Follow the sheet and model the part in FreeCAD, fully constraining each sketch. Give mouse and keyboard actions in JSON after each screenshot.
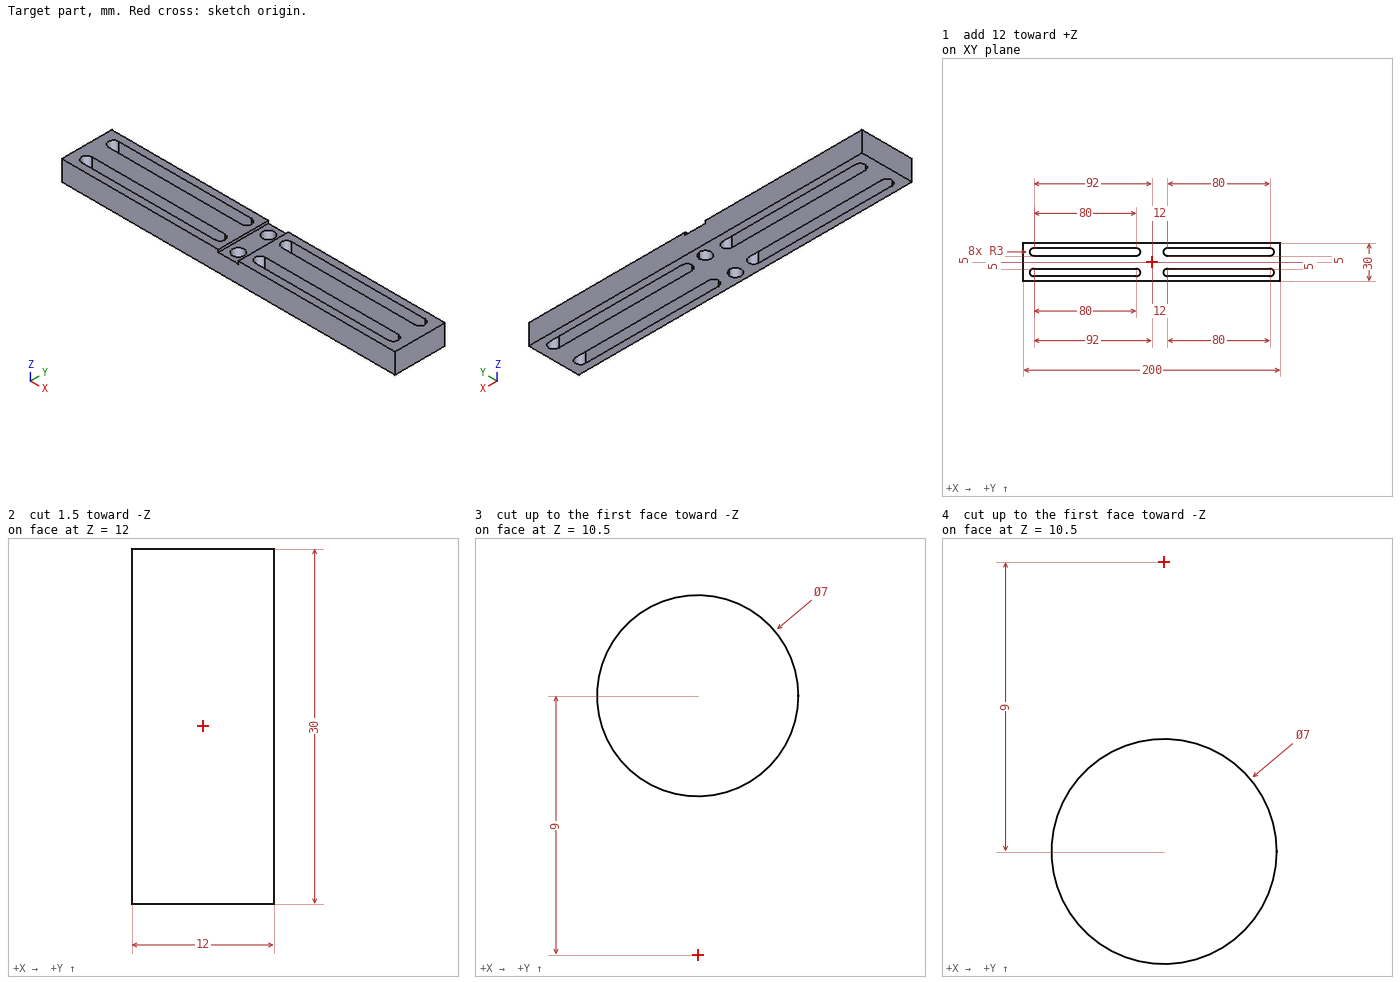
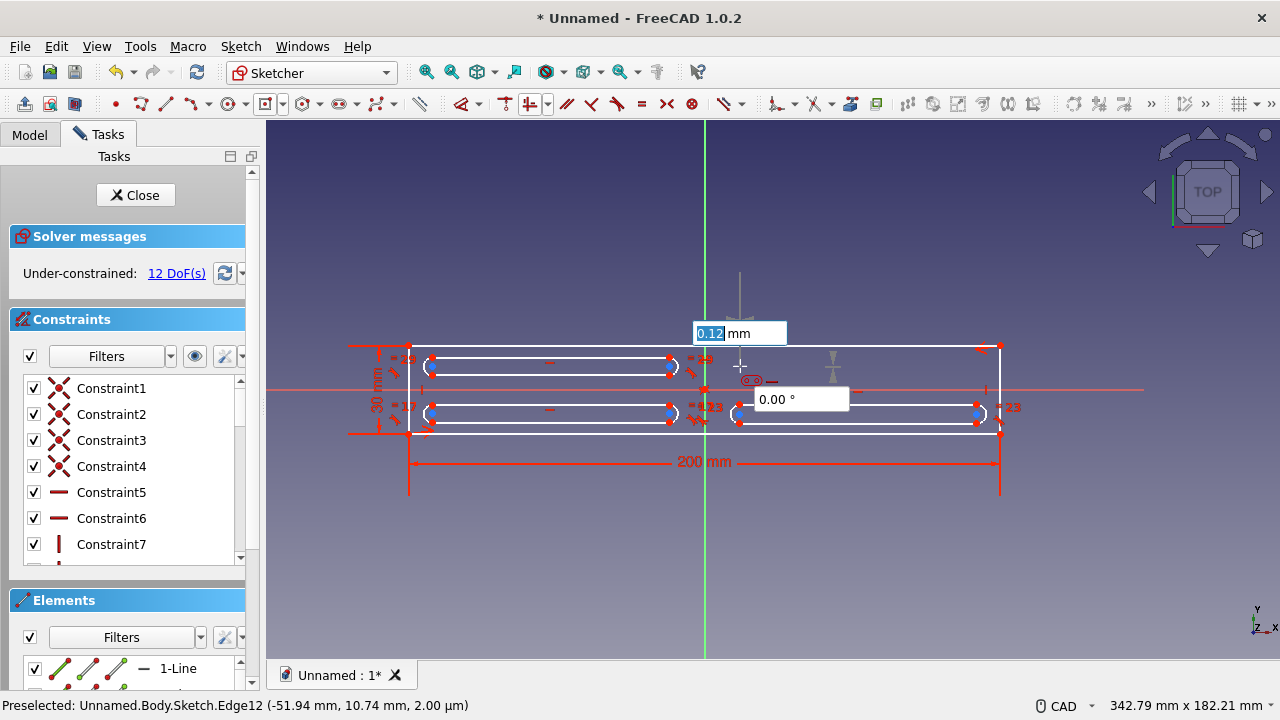
{"action": "left_click", "coordinate": [977, 366]}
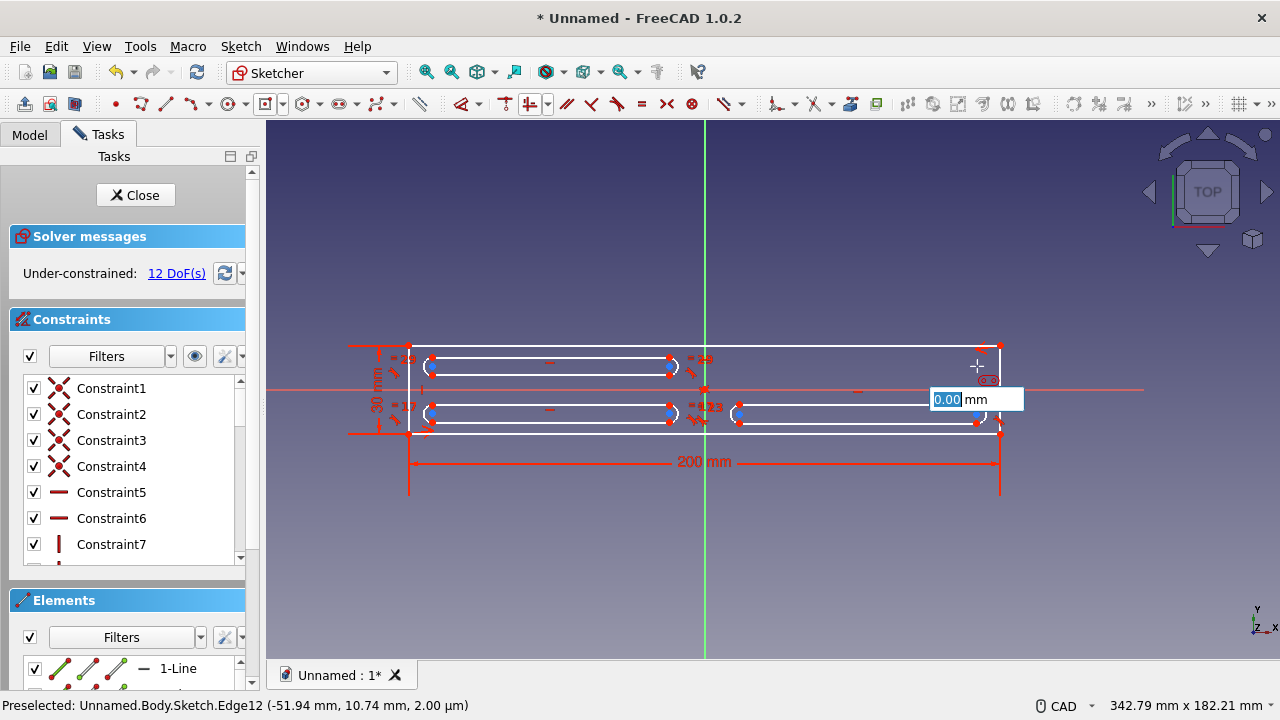
{"action": "scroll", "coordinate": [858, 375], "scroll_direction": "up", "scroll_amount": 3}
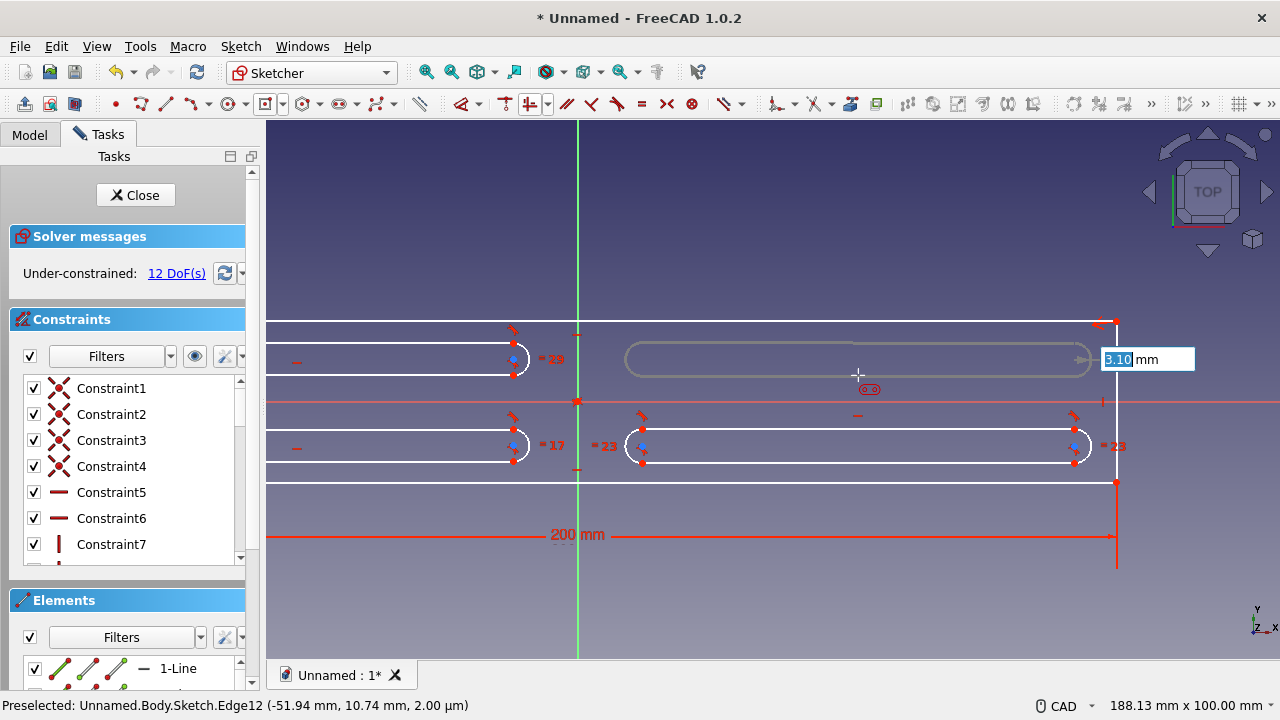
{"action": "left_click", "coordinate": [858, 375]}
{"action": "key", "text": "Escape"}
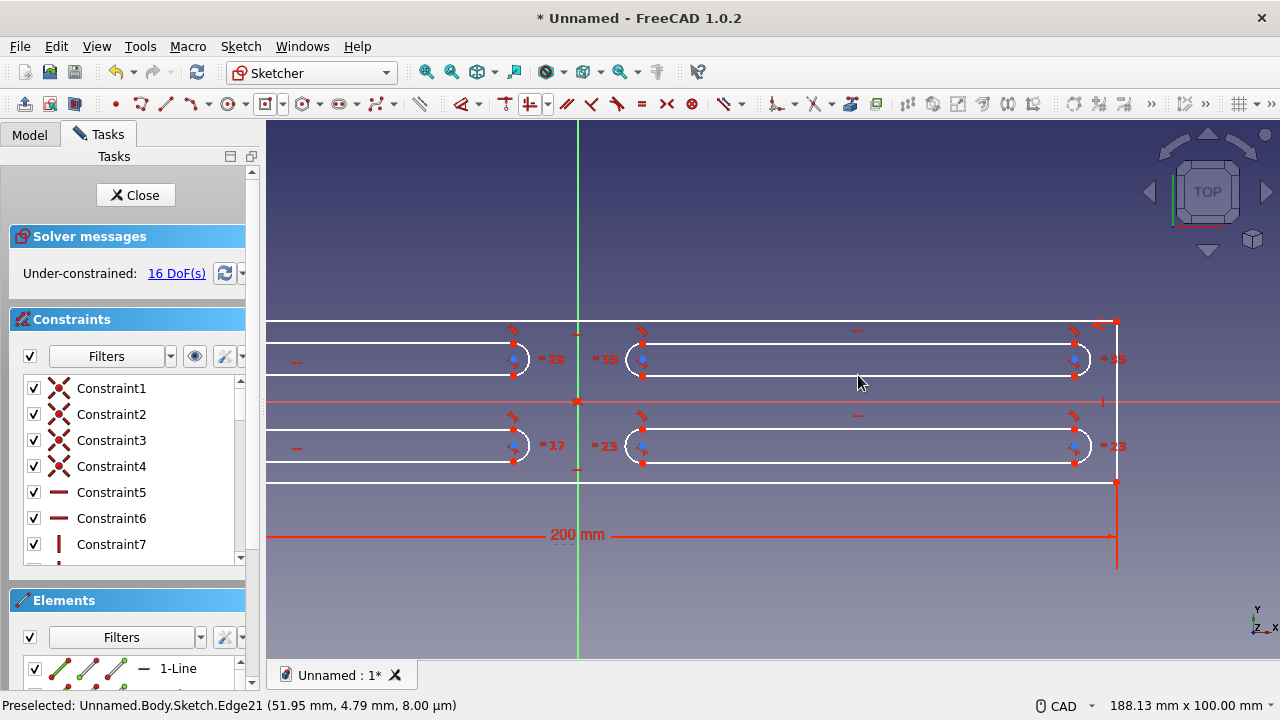
{"action": "scroll", "coordinate": [858, 374], "scroll_direction": "down", "scroll_amount": 3}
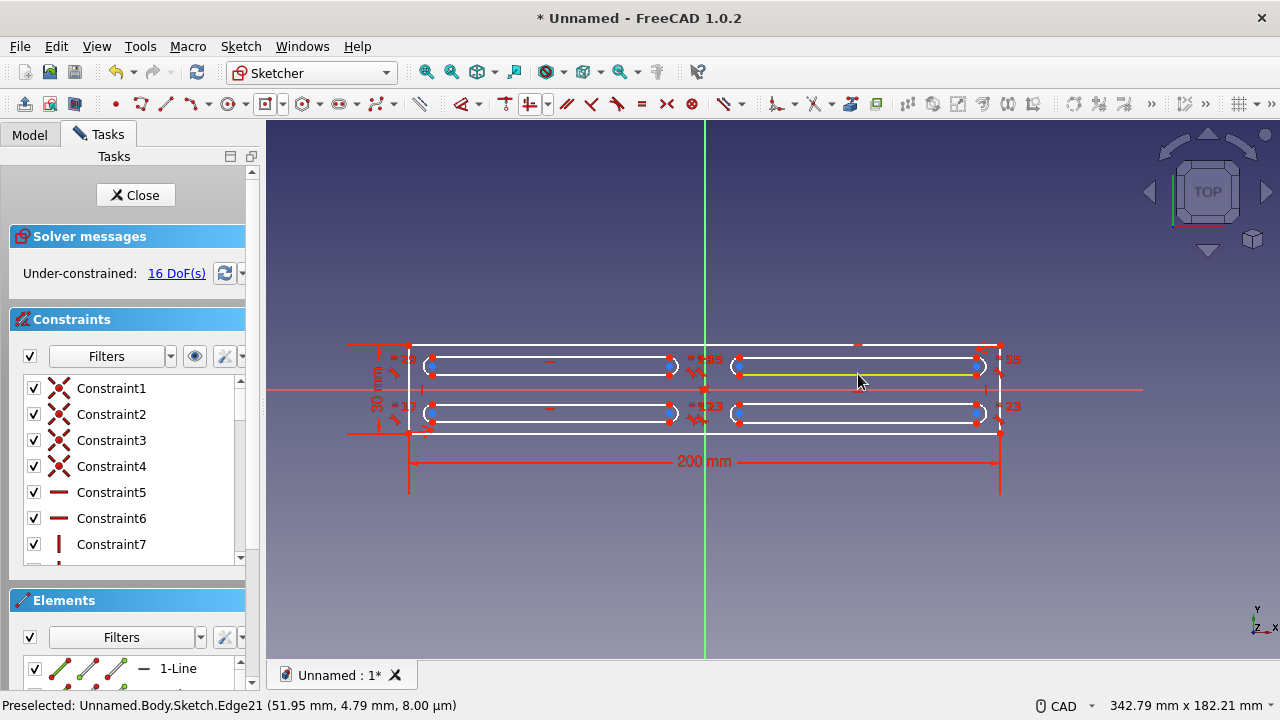
{"action": "scroll", "coordinate": [425, 408], "scroll_direction": "up", "scroll_amount": 3}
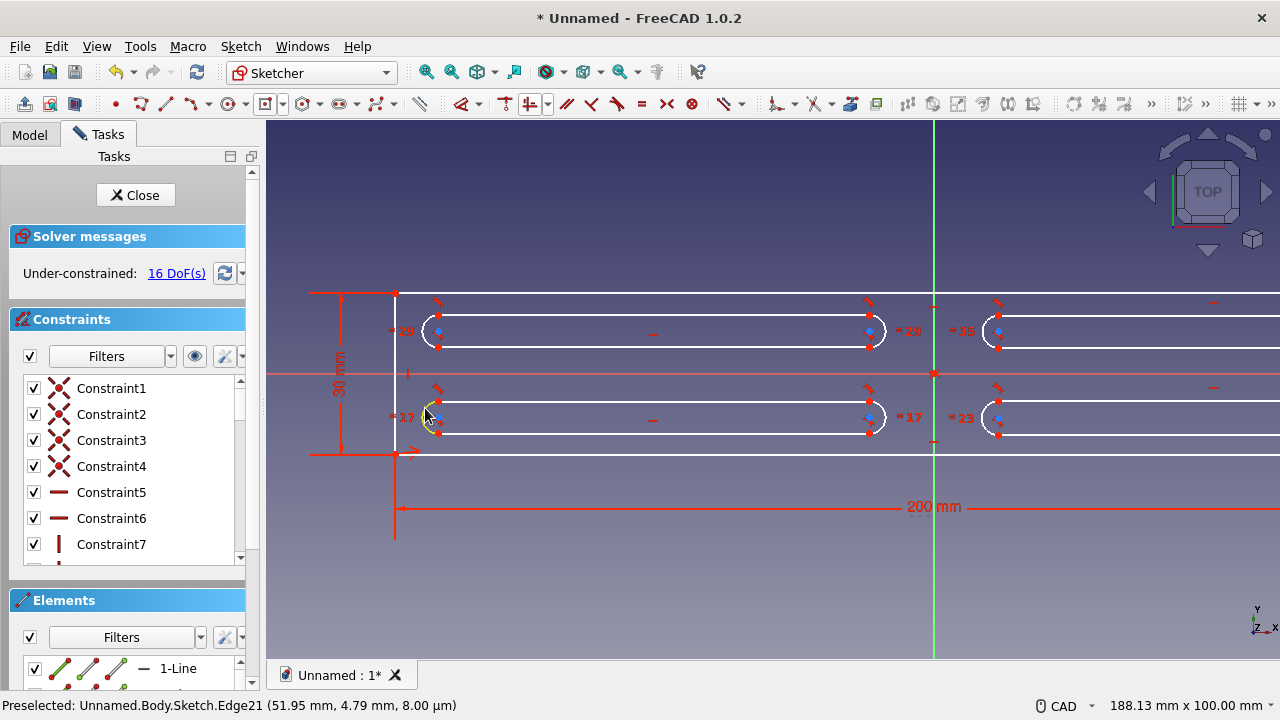
{"action": "left_click", "coordinate": [425, 408]}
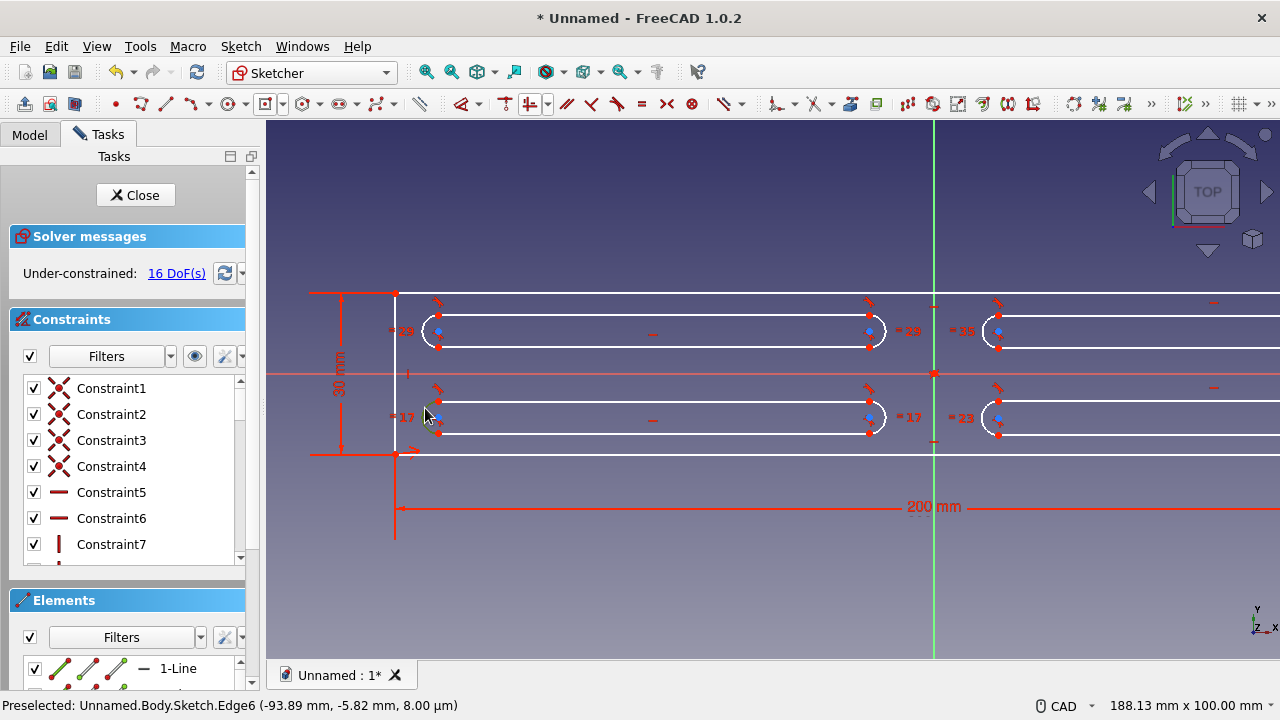
{"action": "left_click", "coordinate": [985, 408]}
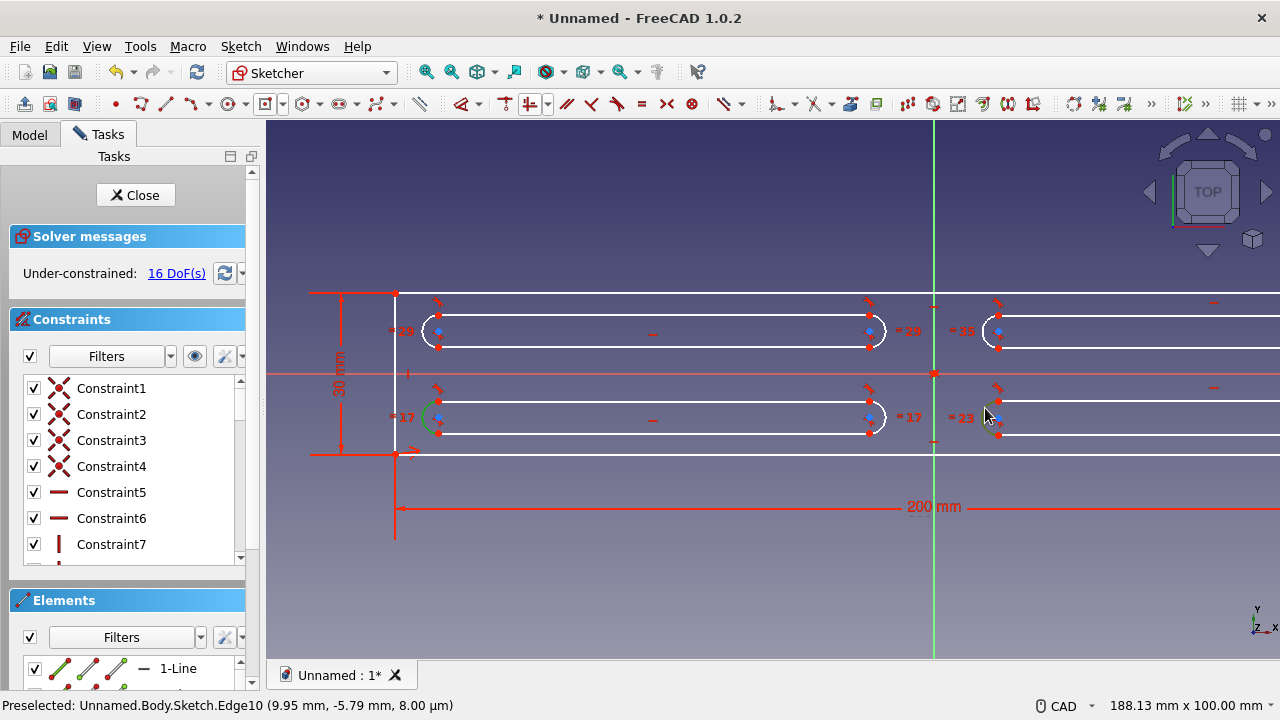
{"action": "left_click", "coordinate": [425, 322]}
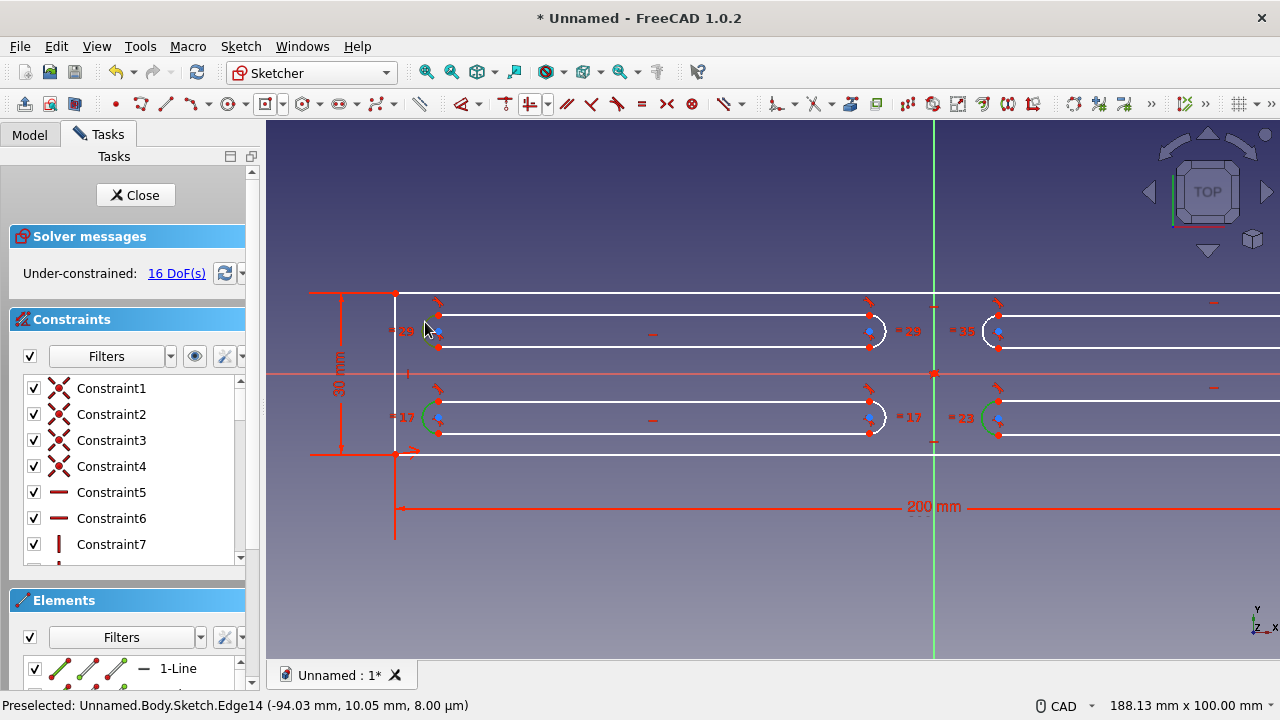
{"action": "left_click", "coordinate": [986, 322]}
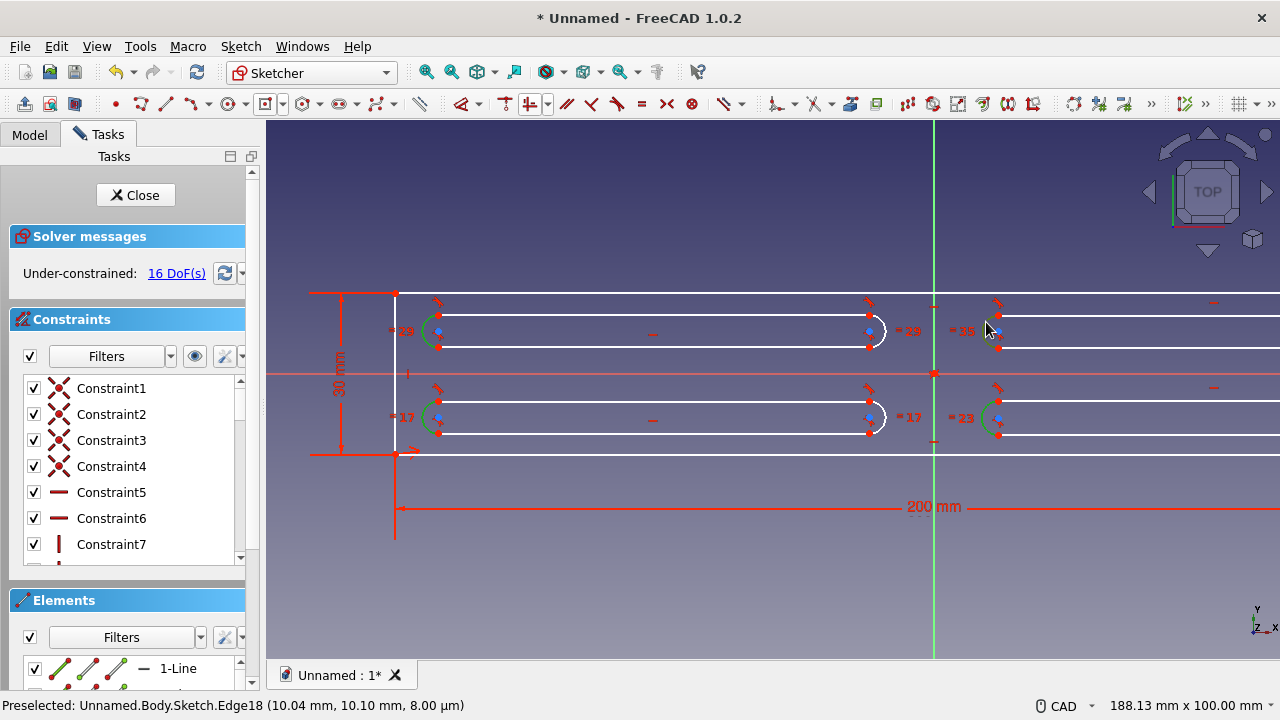
{"action": "left_click", "coordinate": [642, 104]}